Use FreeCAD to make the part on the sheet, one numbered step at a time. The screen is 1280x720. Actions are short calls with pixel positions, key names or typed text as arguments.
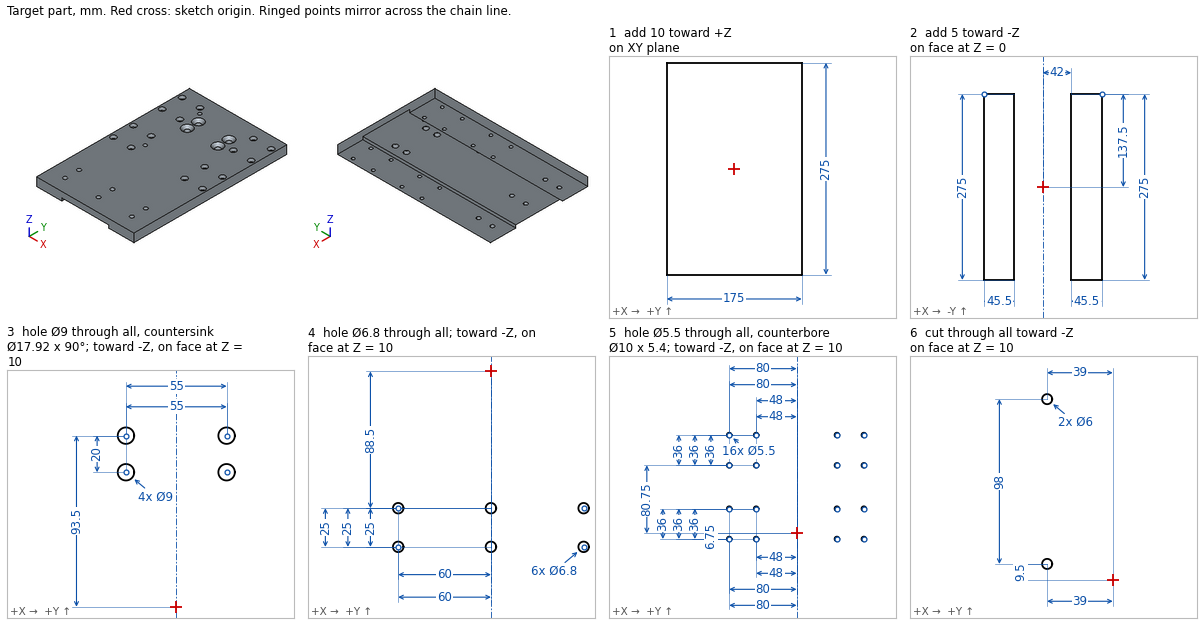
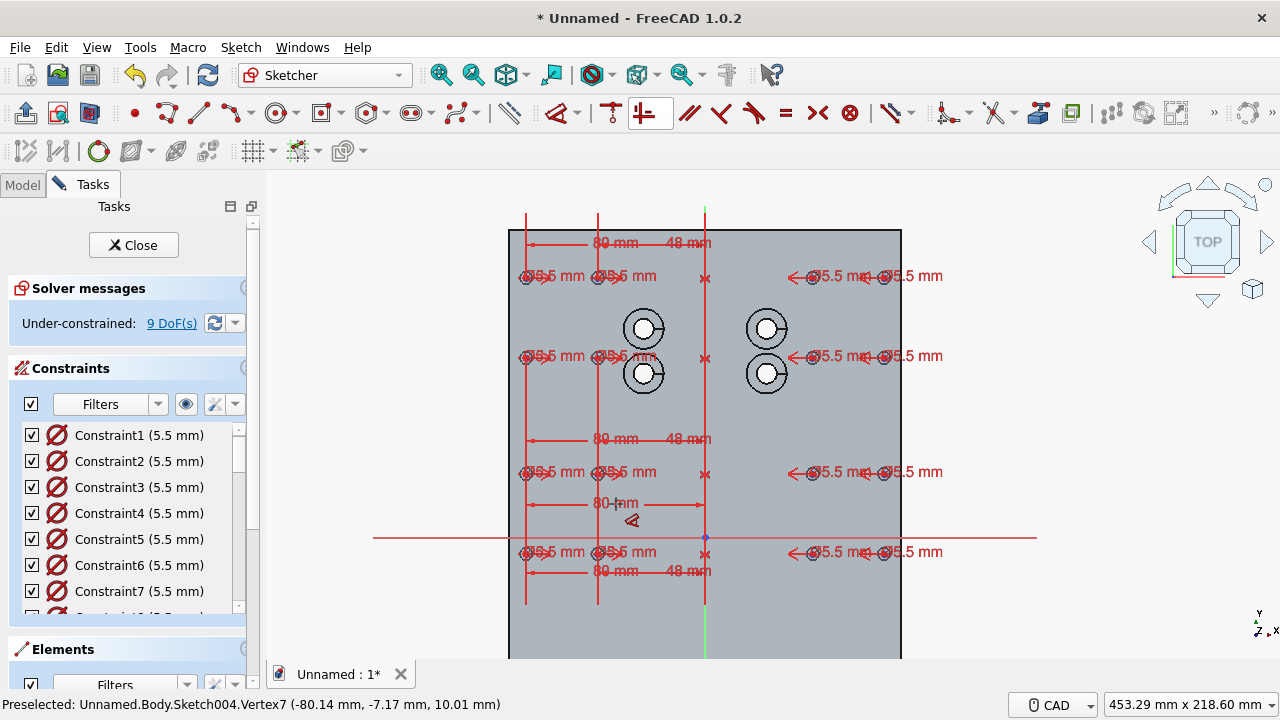
click(598, 554)
click(689, 504)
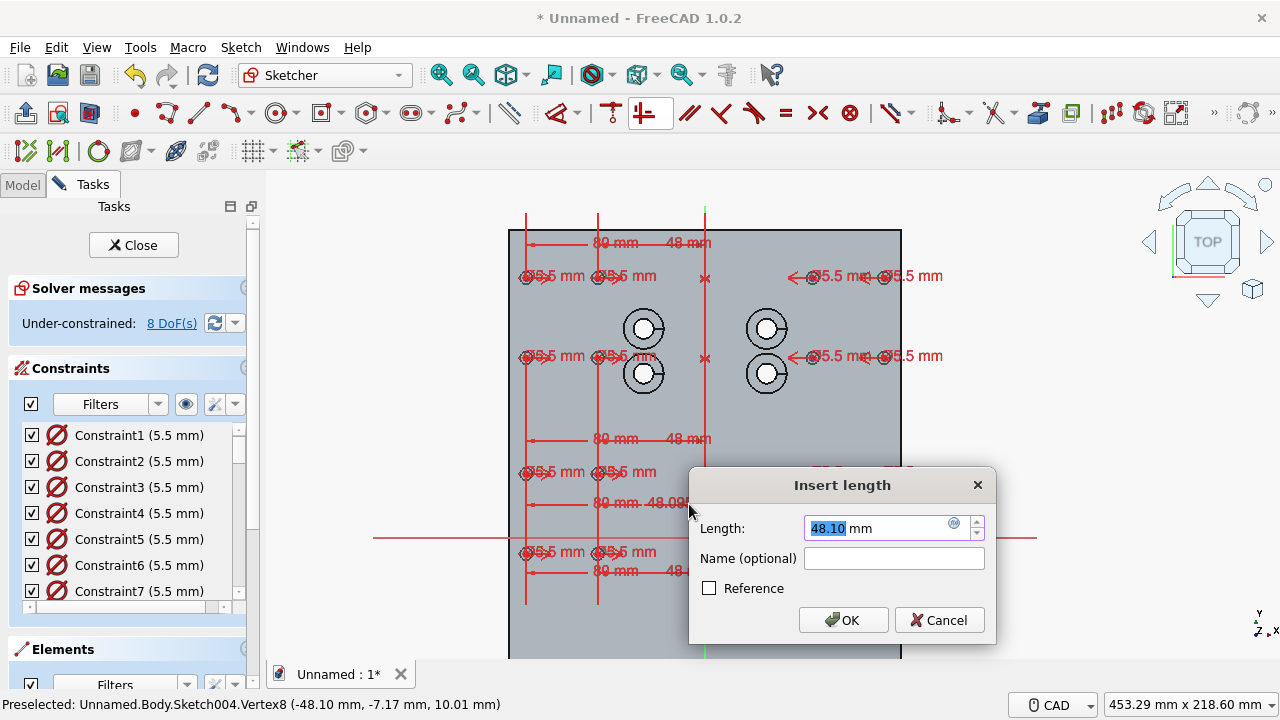
text(48)
key(Return)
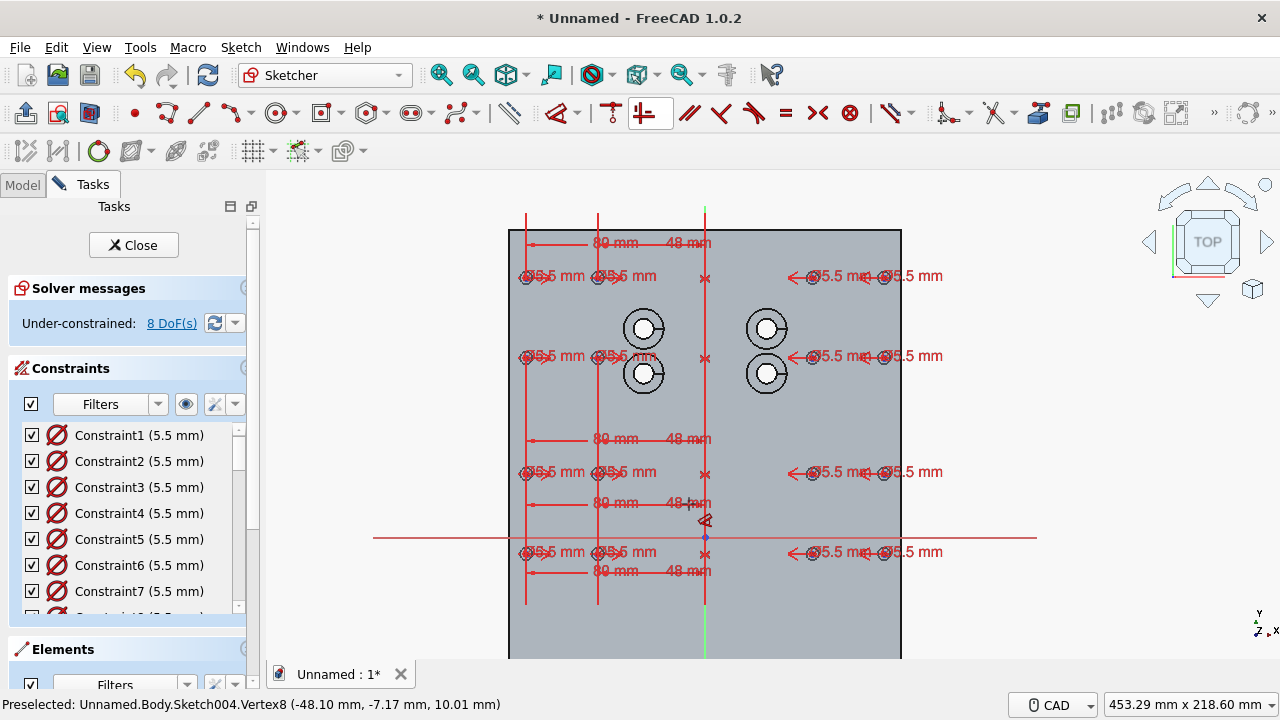
click(526, 278)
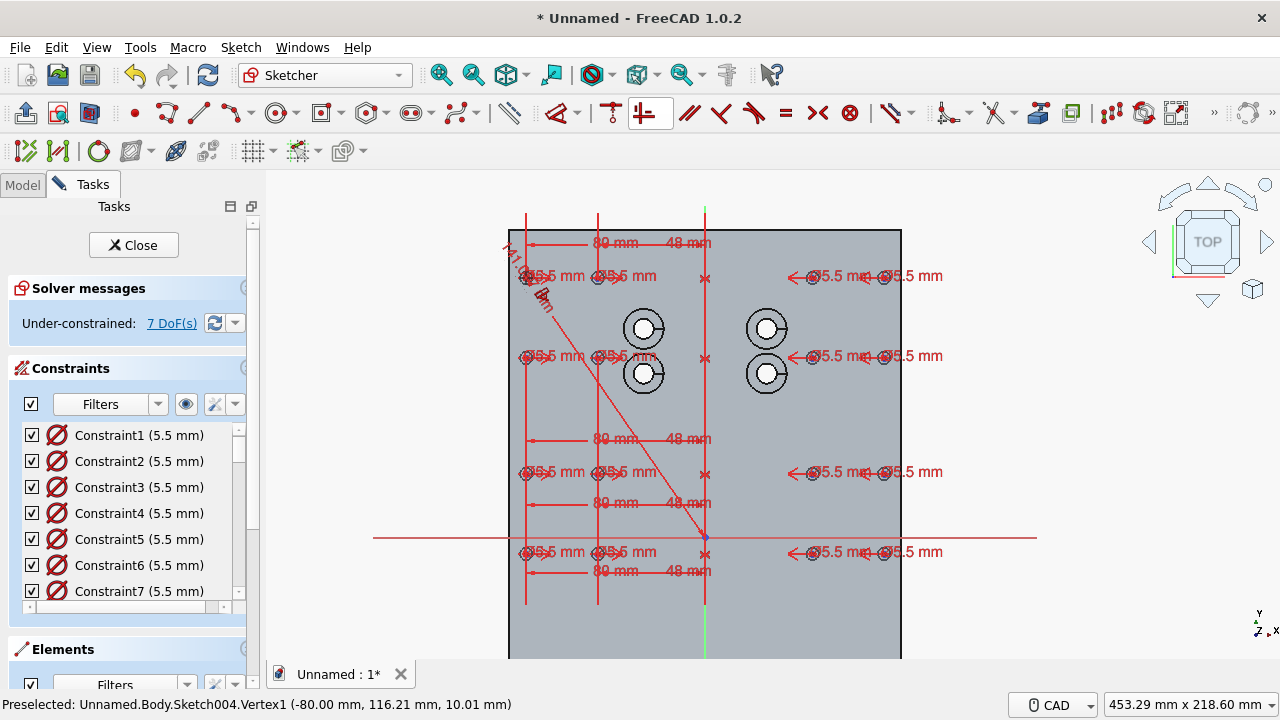
click(526, 358)
click(492, 318)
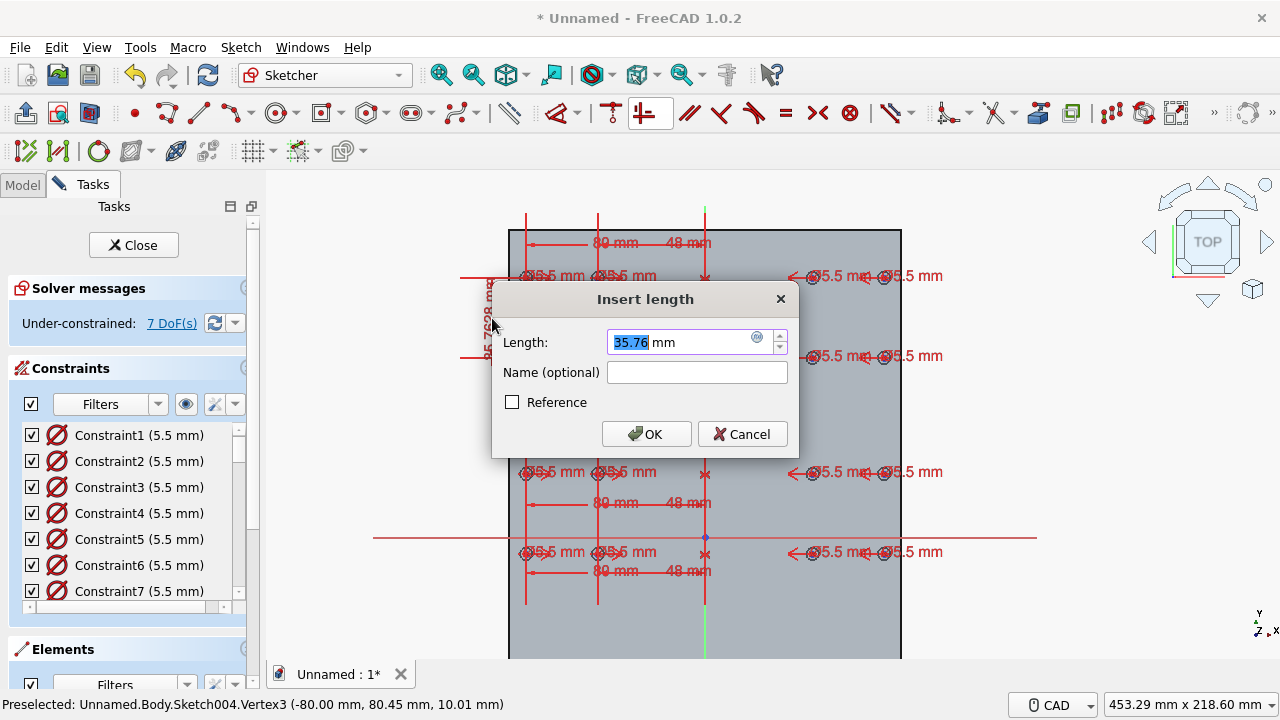
text(36)
key(Return)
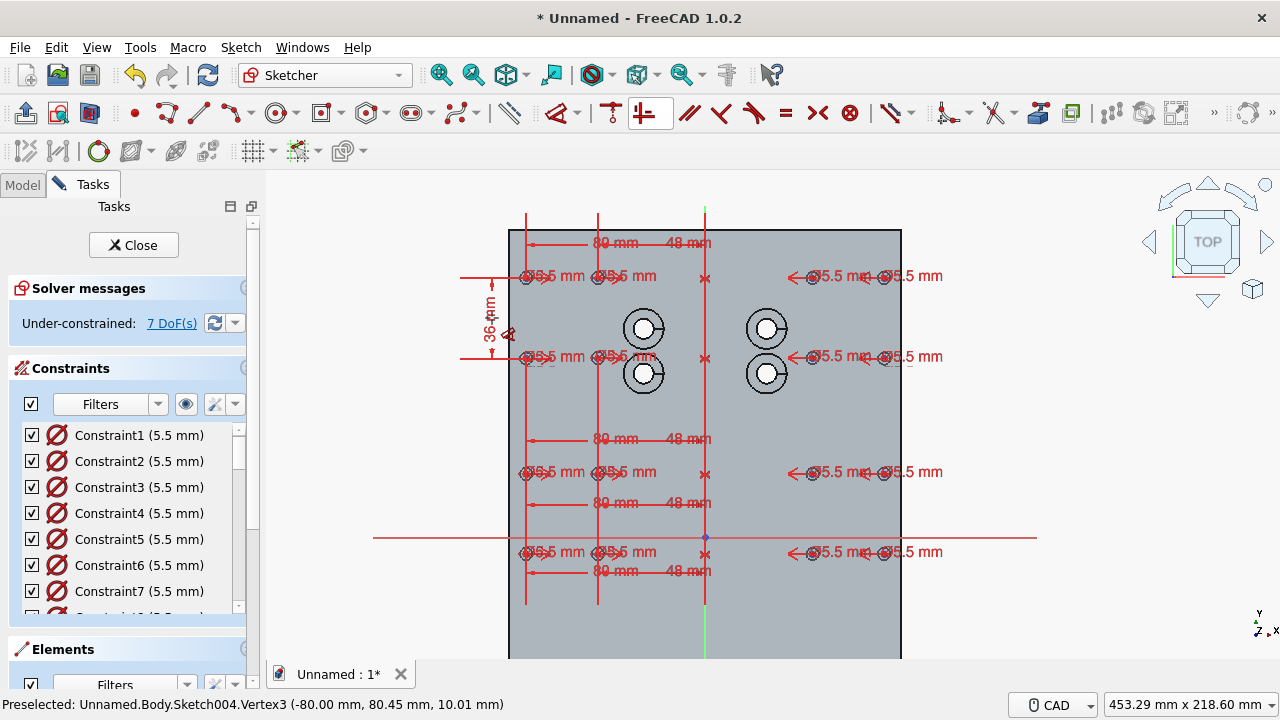
click(598, 278)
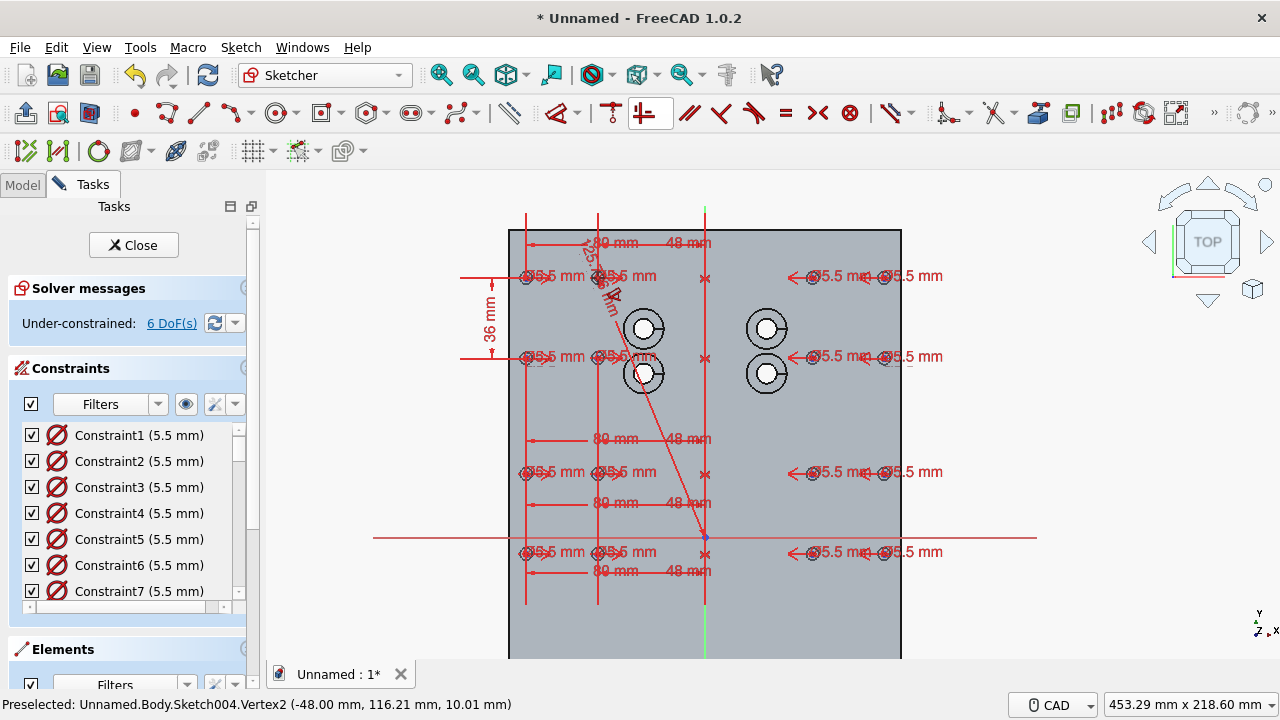
click(526, 359)
click(492, 290)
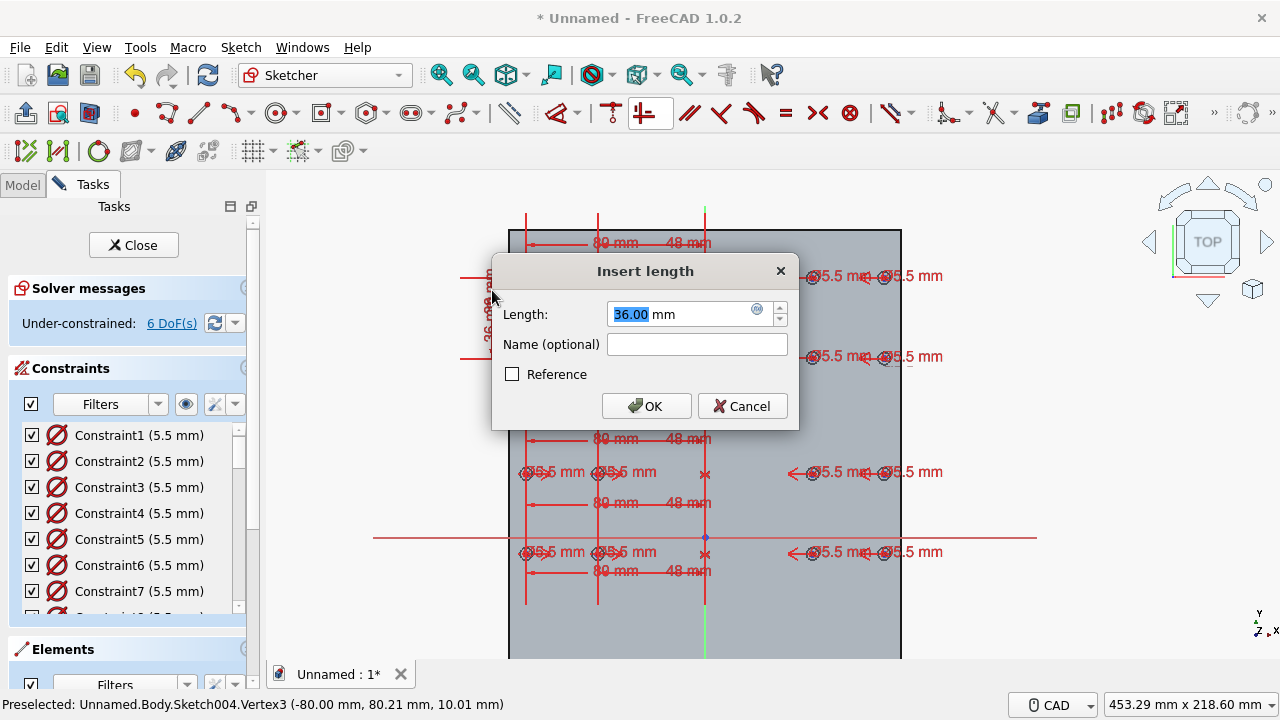
text(36)
key(Return)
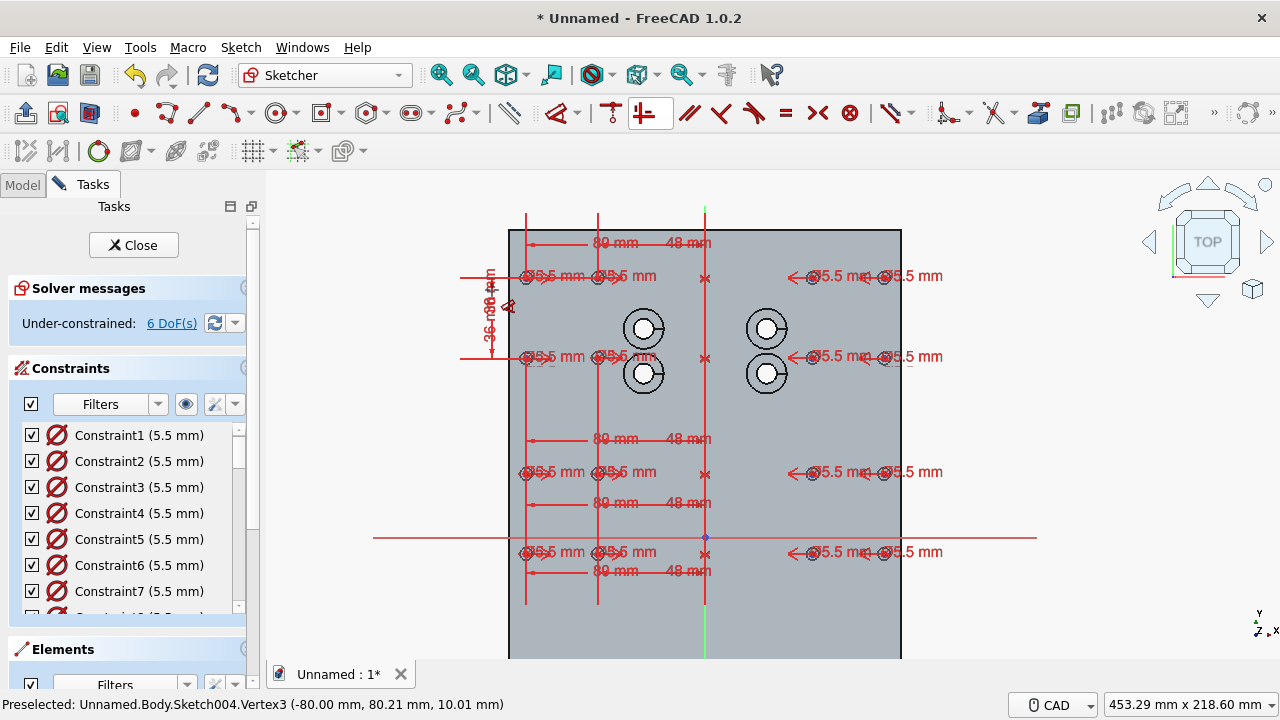
click(598, 278)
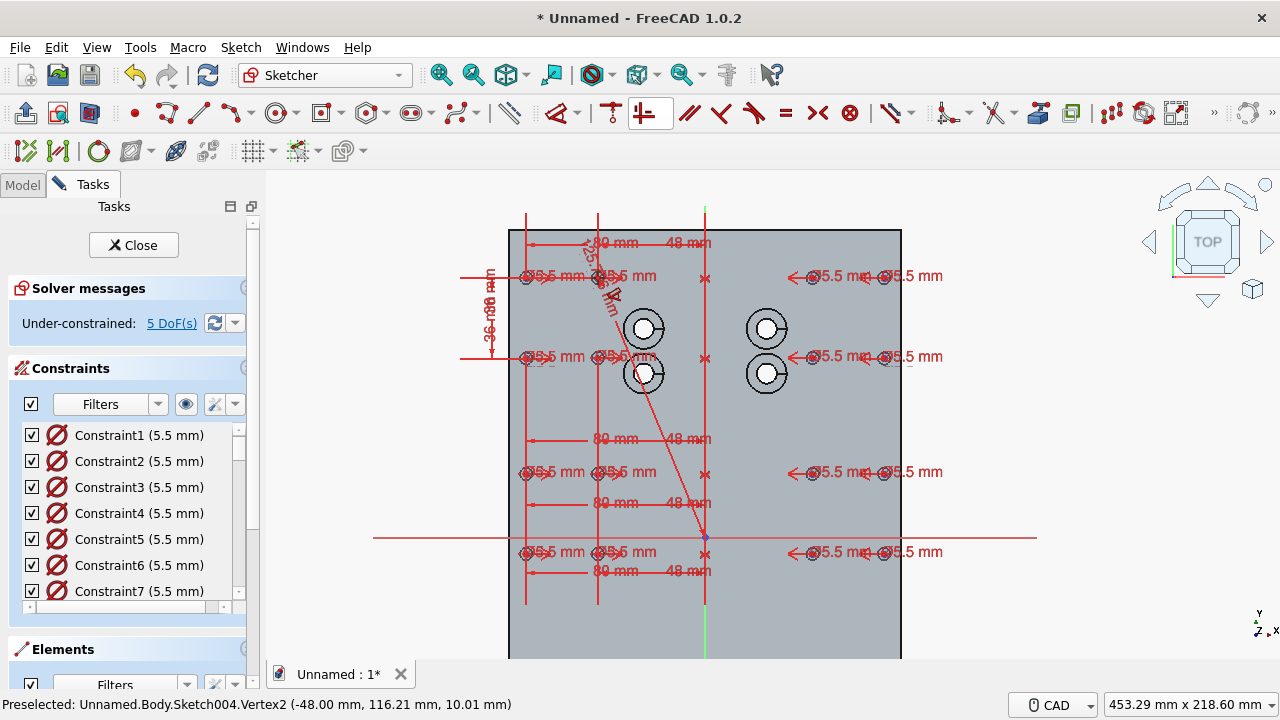
click(598, 358)
click(564, 318)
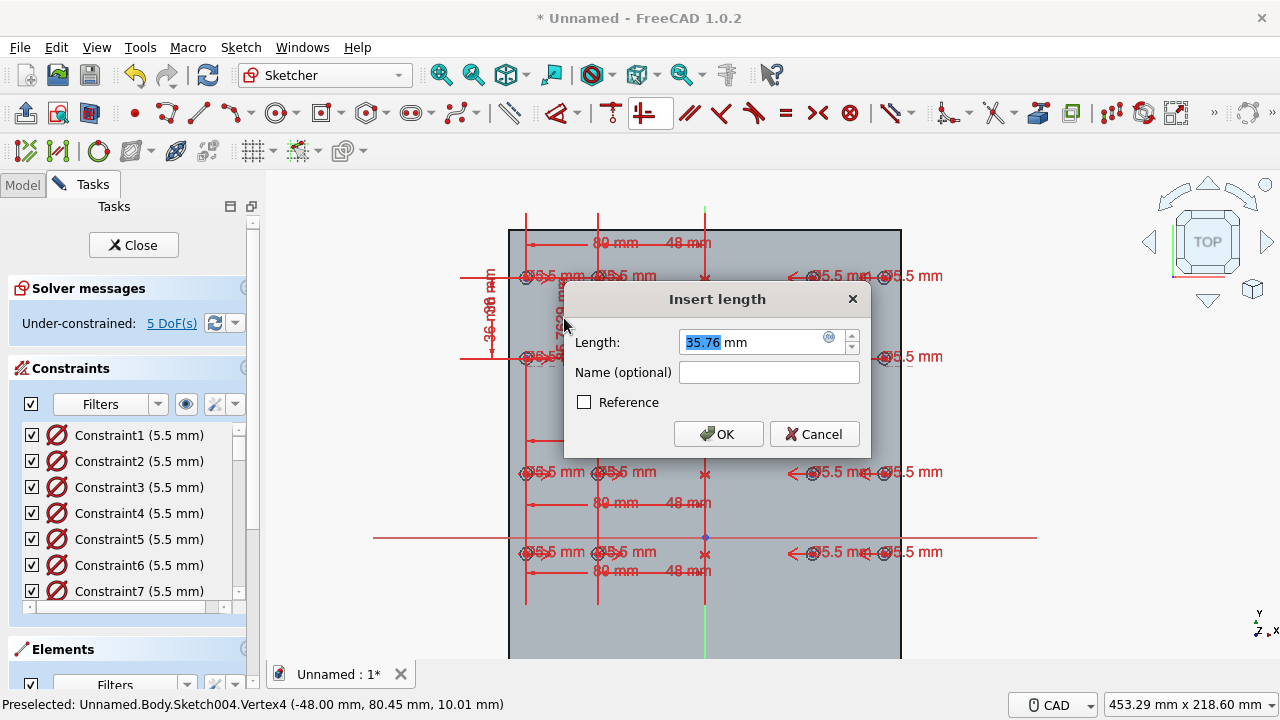
text(36)
key(Return)